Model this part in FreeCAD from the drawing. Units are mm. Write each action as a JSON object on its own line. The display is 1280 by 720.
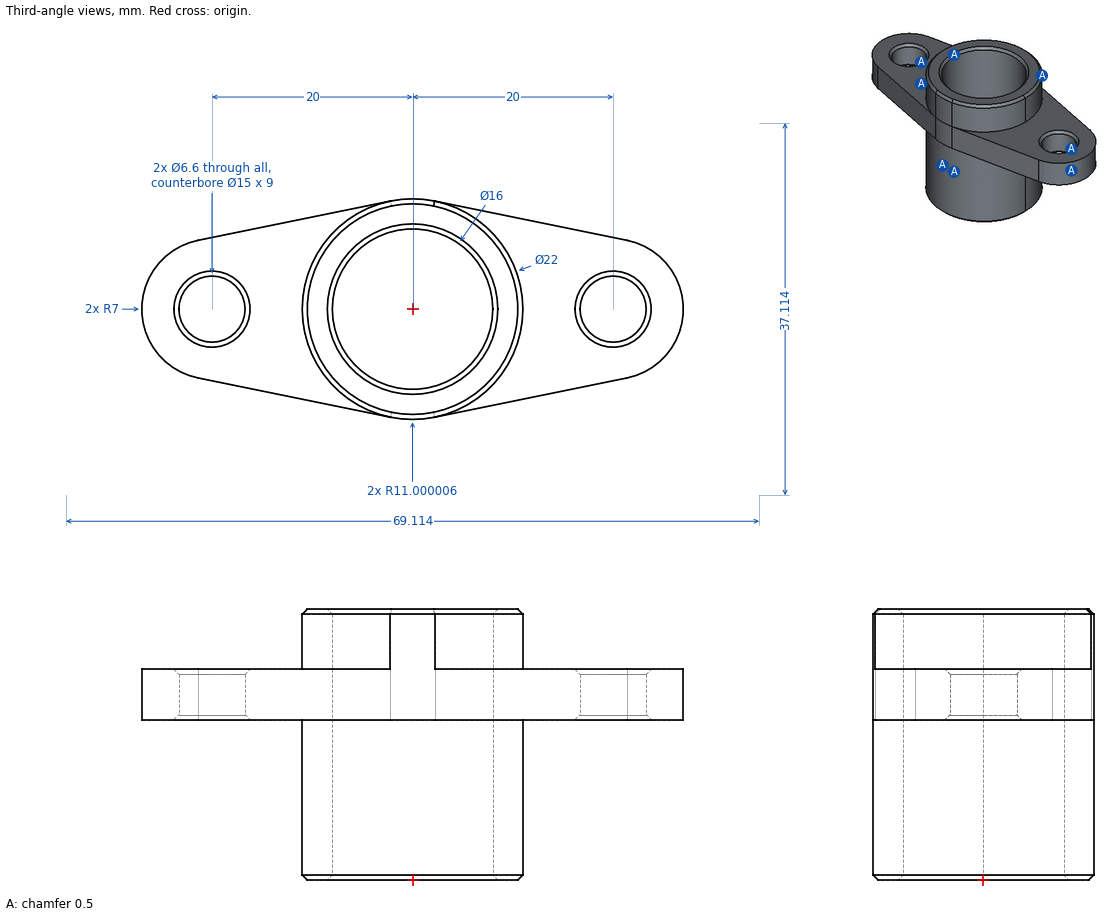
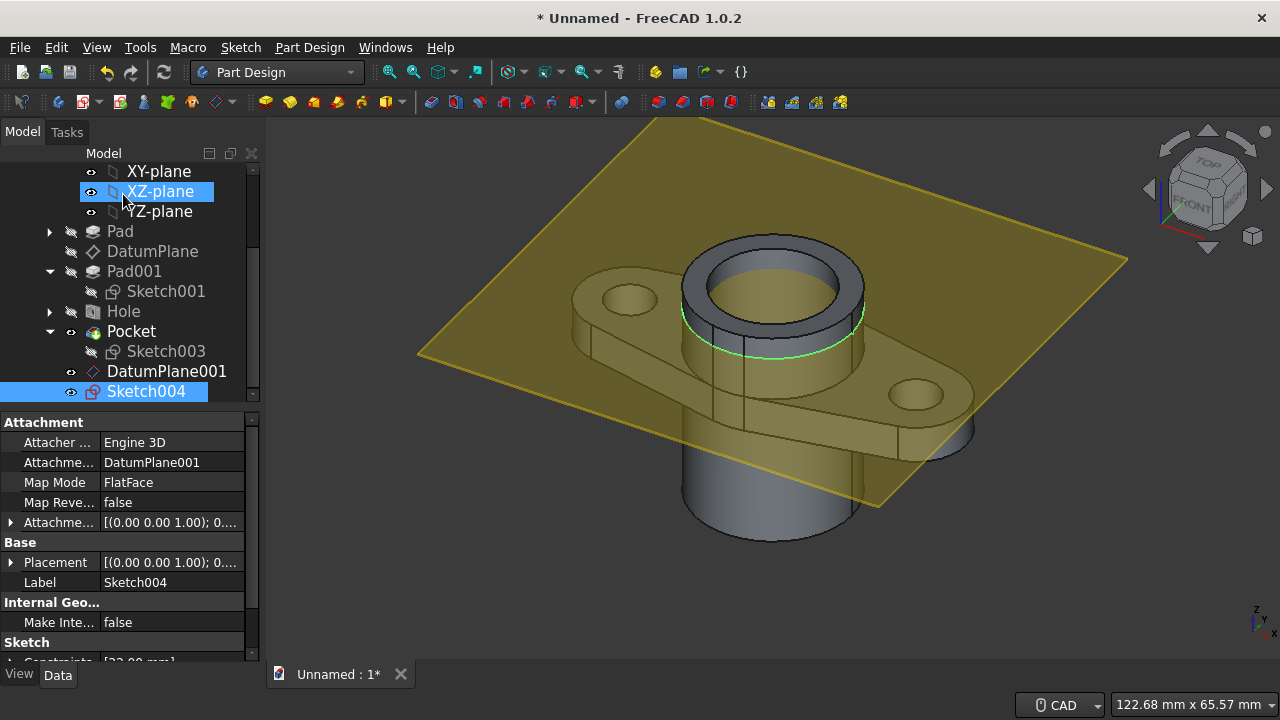
{"action": "left_click", "coordinate": [432, 102]}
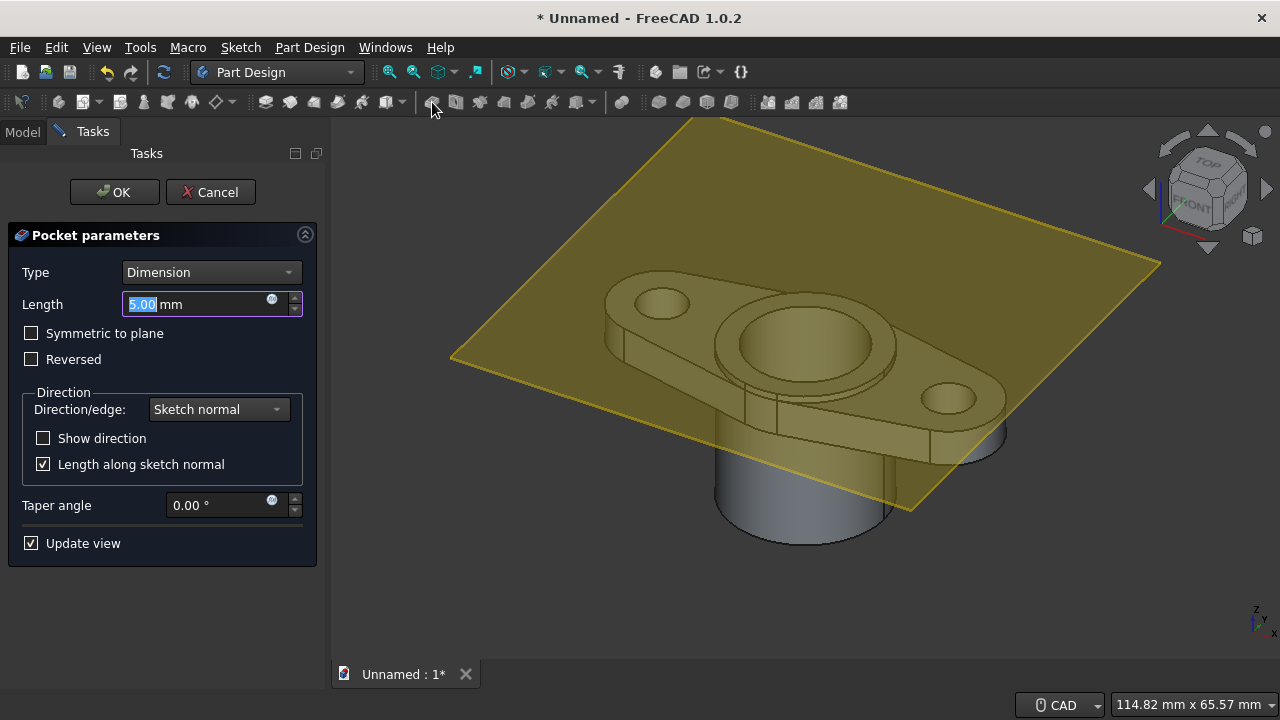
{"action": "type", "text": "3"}
{"action": "key", "text": "Tab"}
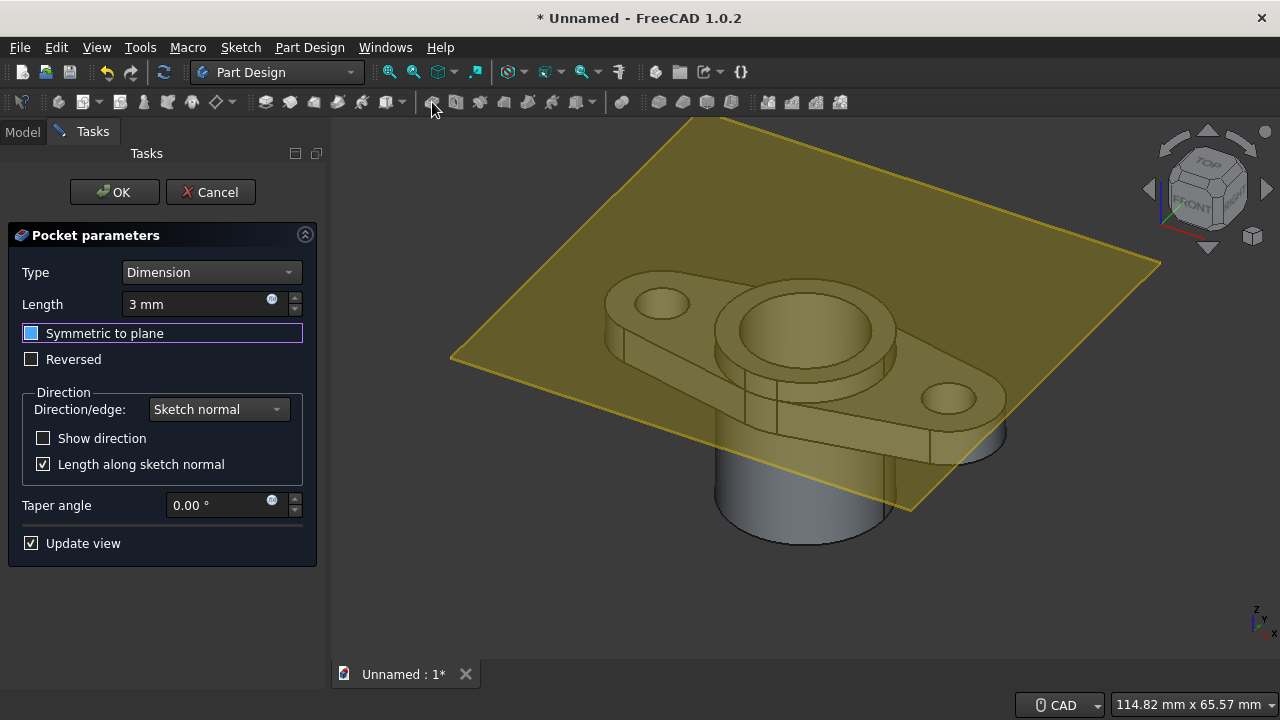
{"action": "left_click", "coordinate": [30, 359]}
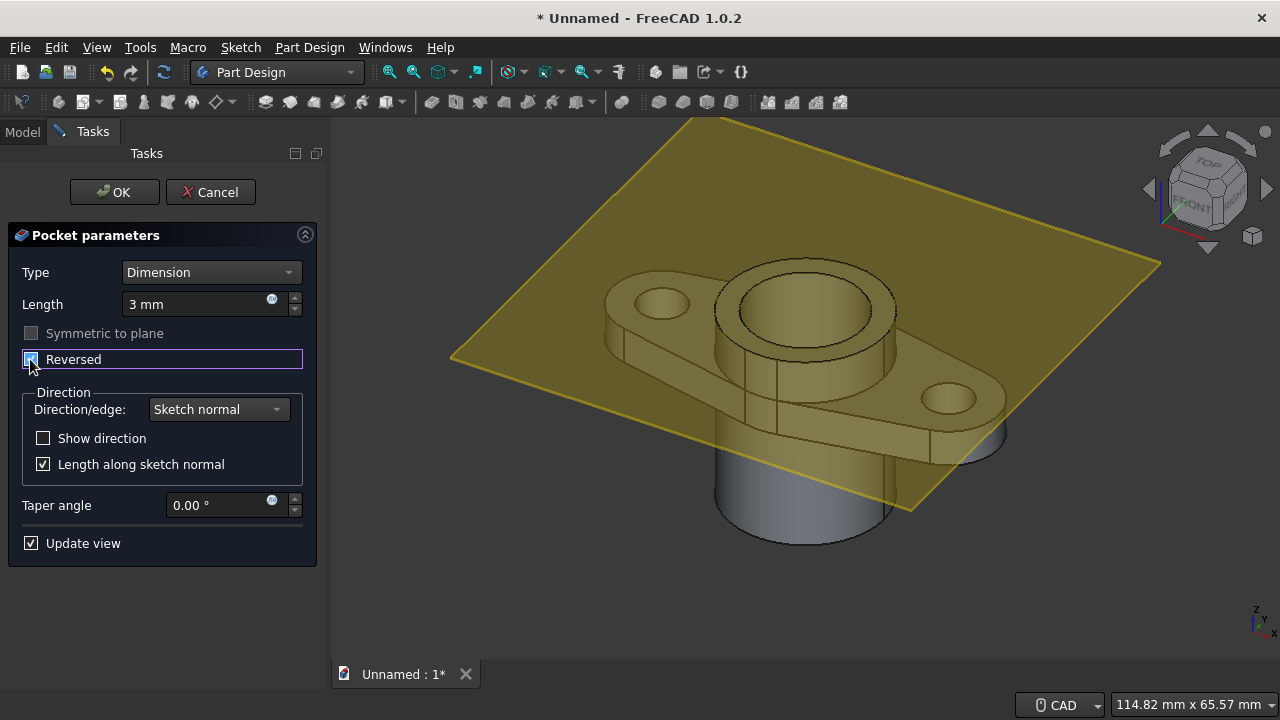
{"action": "left_click", "coordinate": [115, 192]}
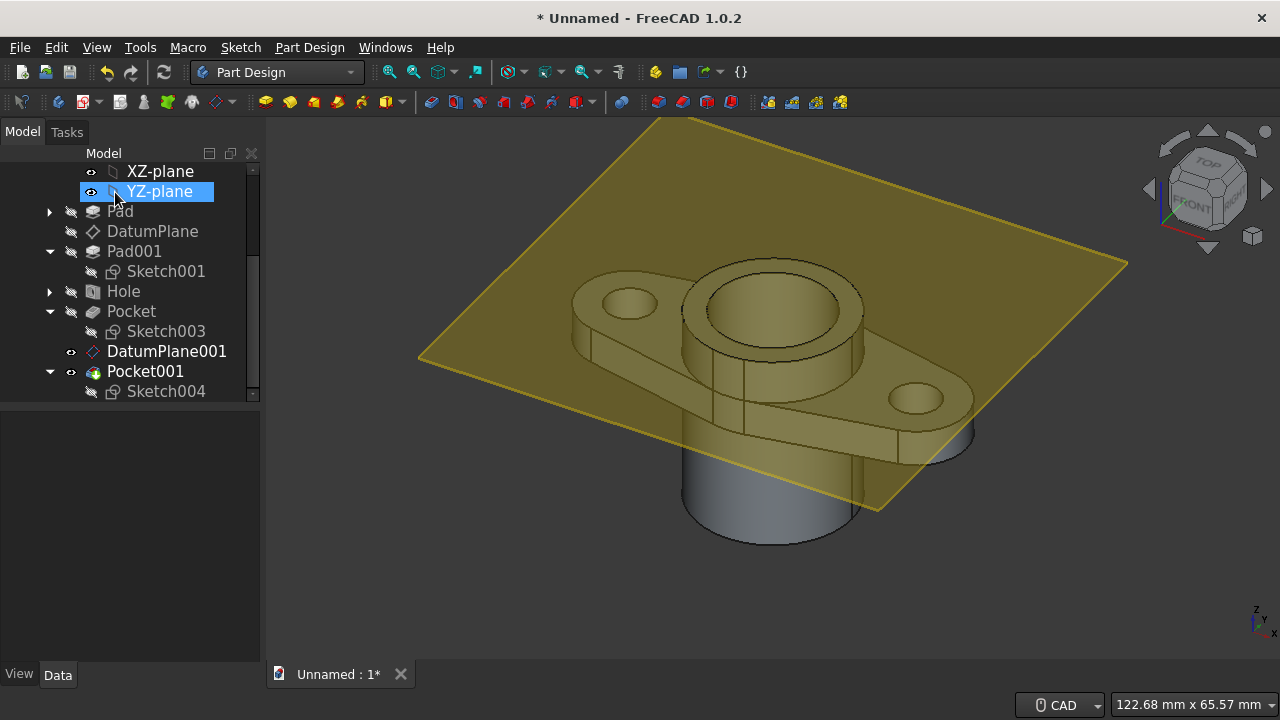
{"action": "left_click", "coordinate": [116, 352]}
{"action": "key", "text": "space"}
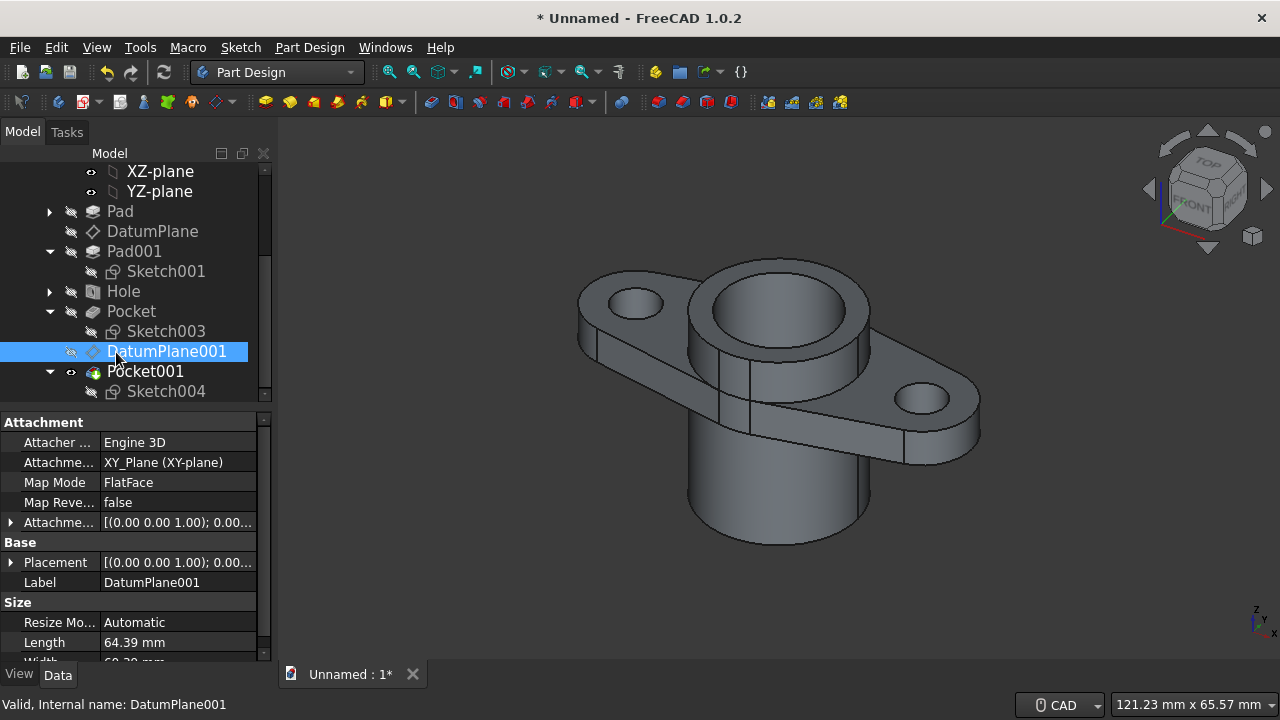
{"action": "left_click", "coordinate": [869, 315]}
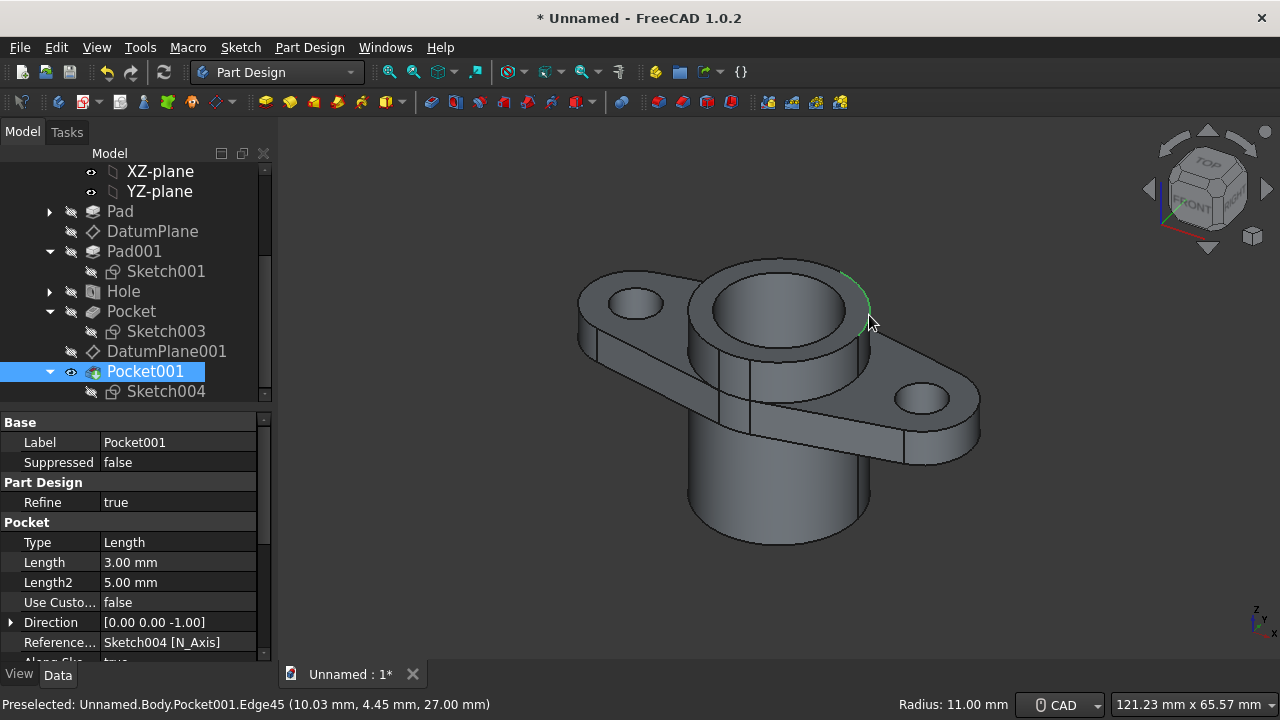
{"action": "left_click", "coordinate": [722, 291], "text": "ctrl"}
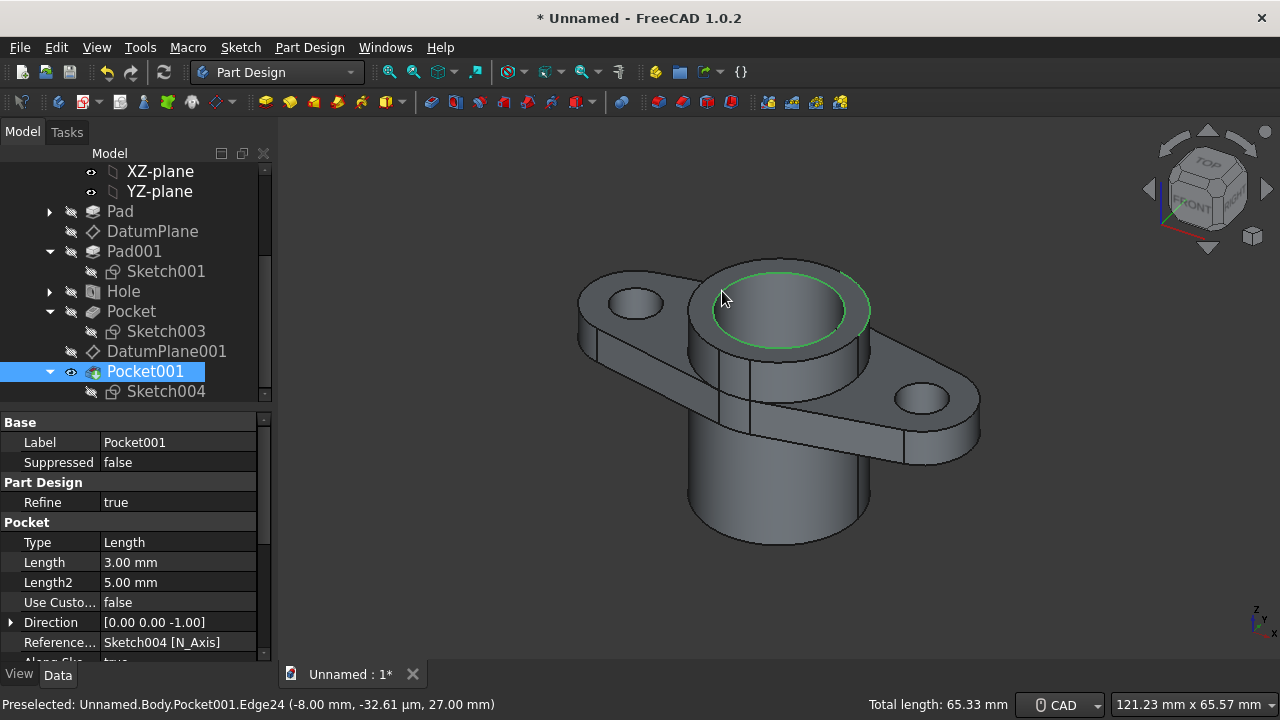
{"action": "left_click", "coordinate": [899, 390], "text": "ctrl"}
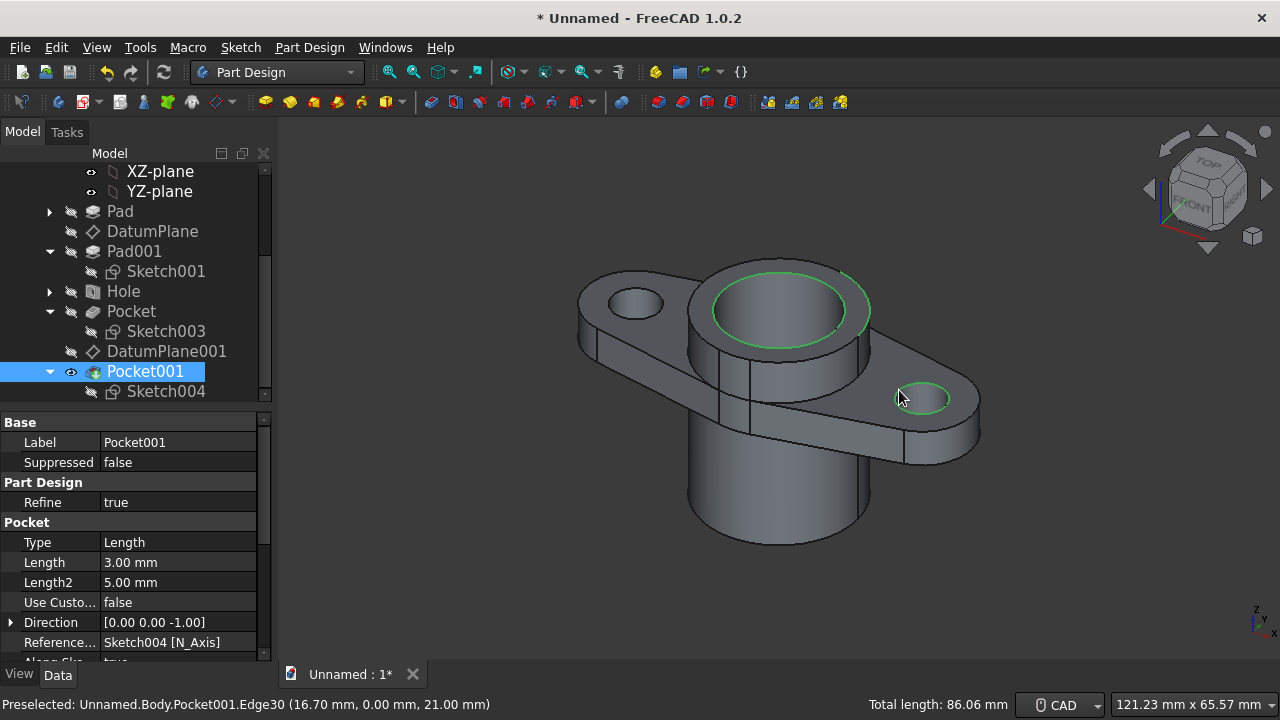
{"action": "left_click", "coordinate": [612, 295], "text": "ctrl"}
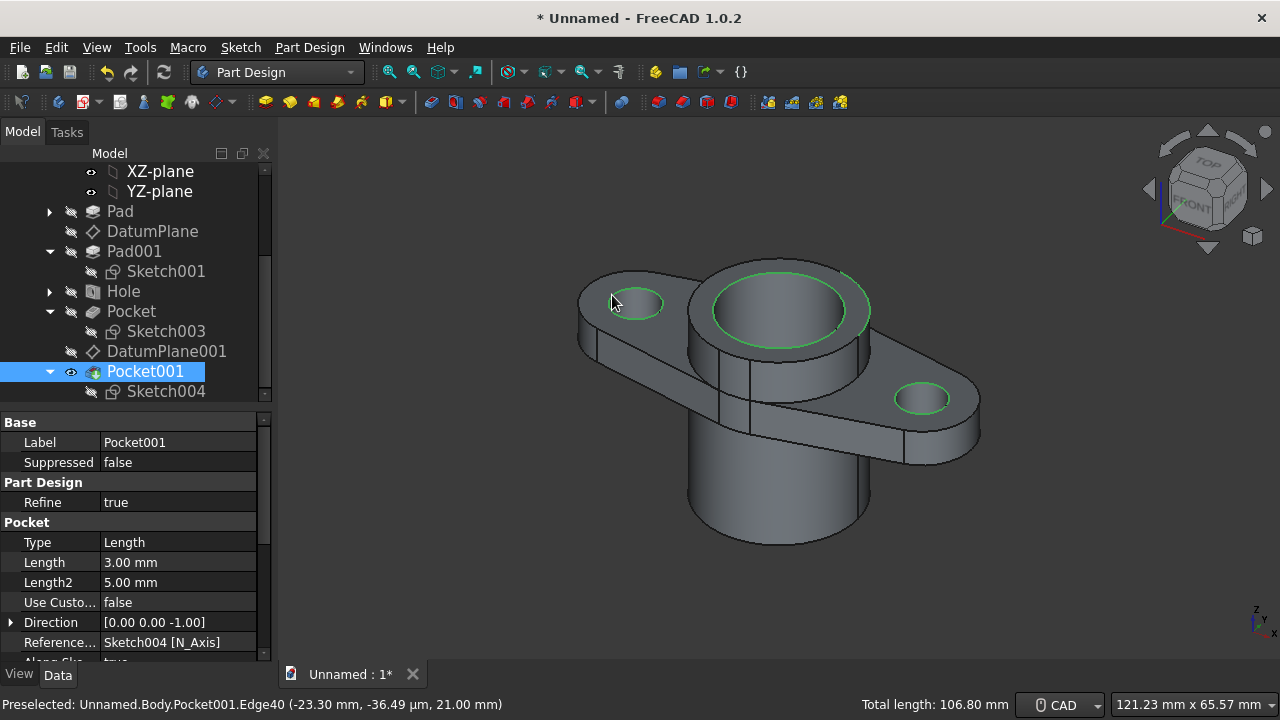
{"action": "key", "text": "0"}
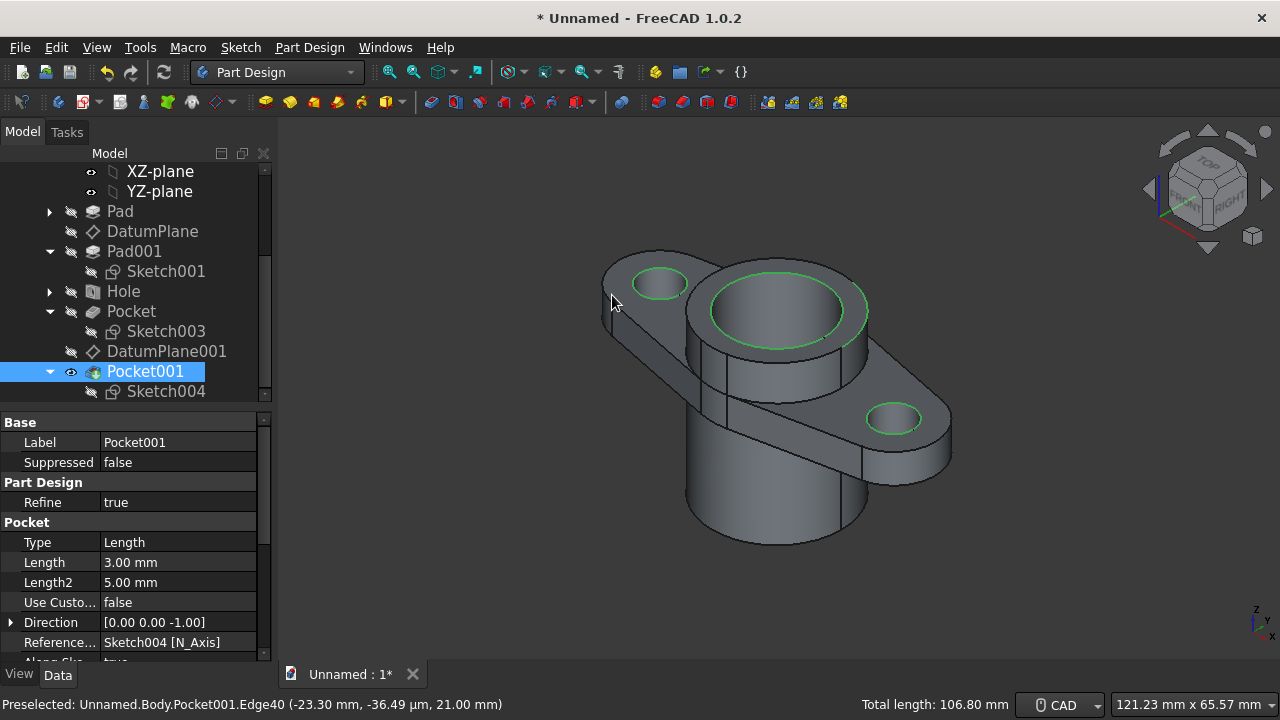
{"action": "key", "text": "2"}